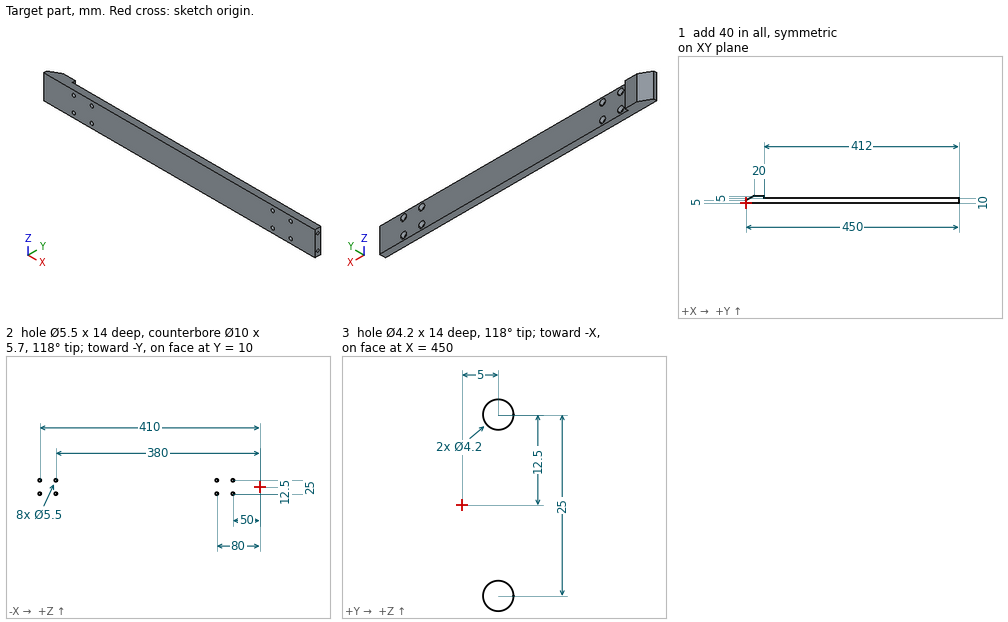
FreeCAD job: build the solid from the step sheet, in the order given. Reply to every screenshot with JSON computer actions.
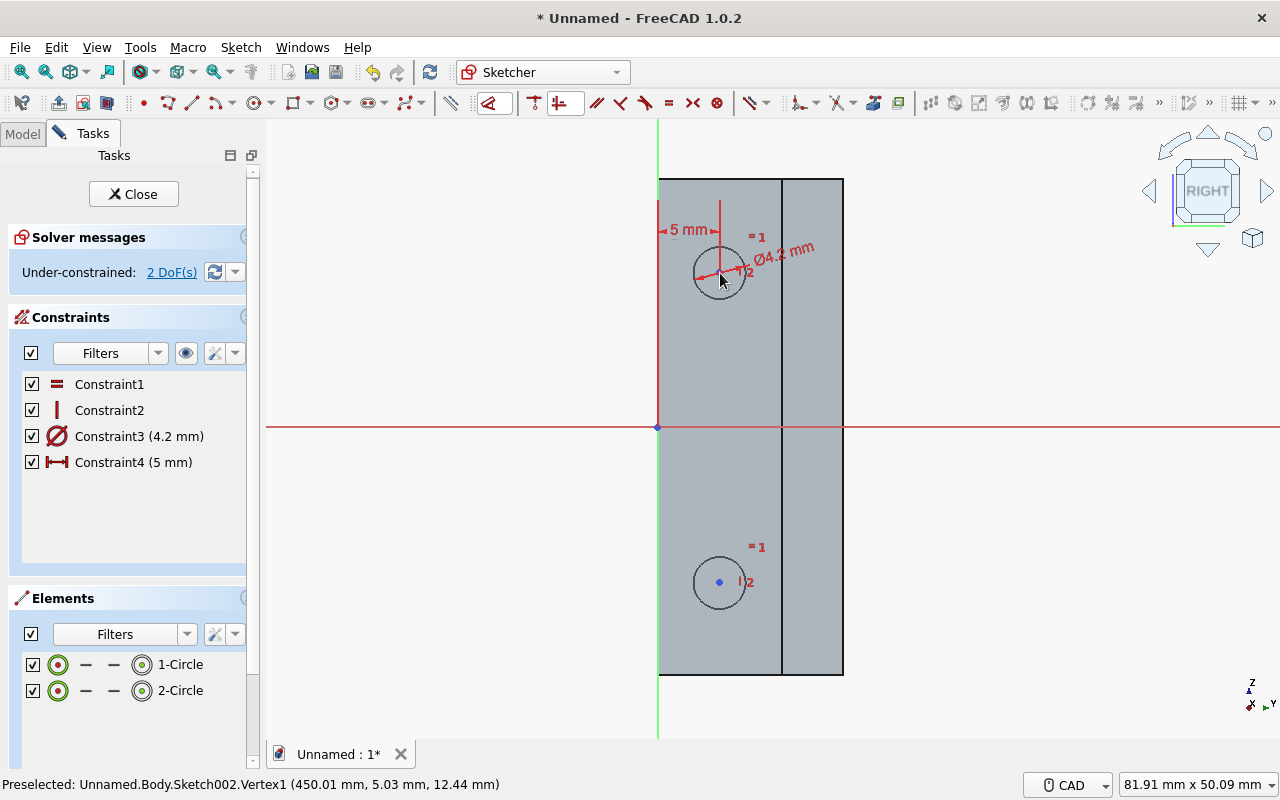
{"action": "left_click", "coordinate": [720, 273]}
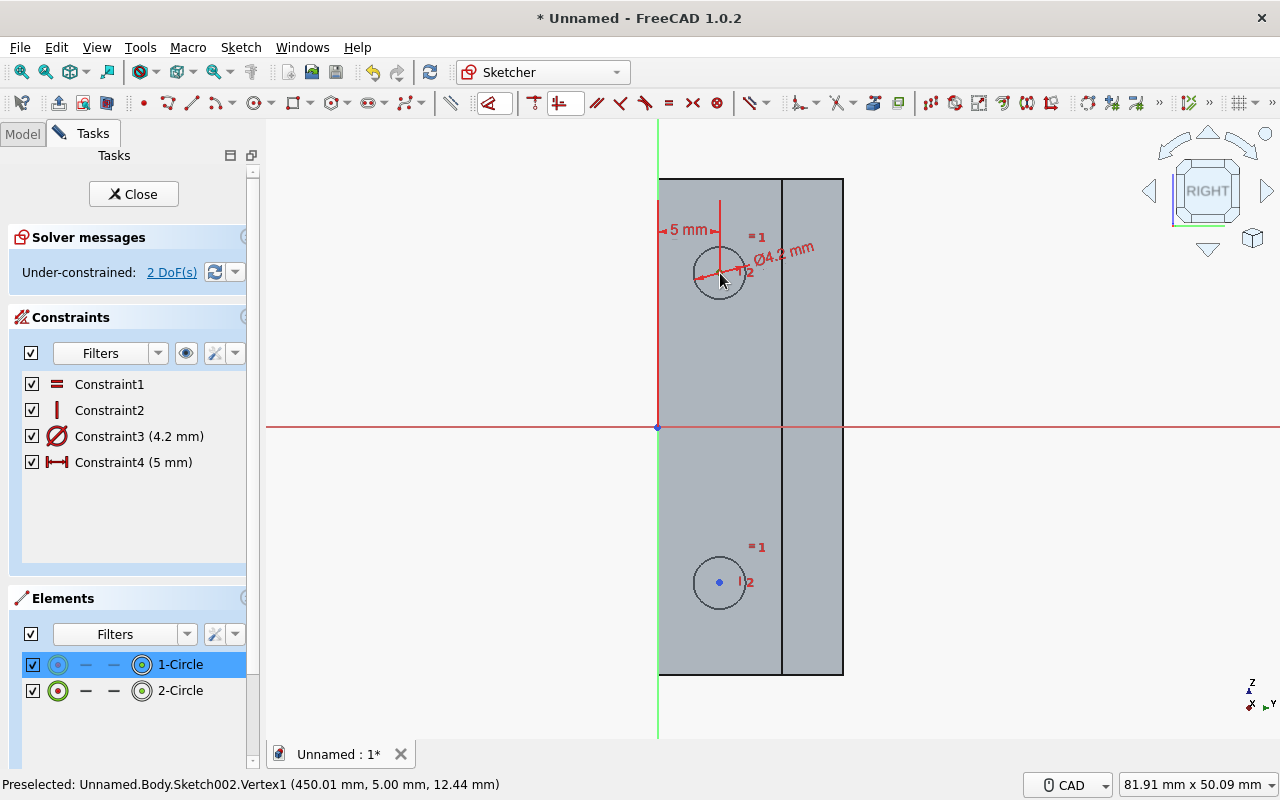
{"action": "left_click", "coordinate": [720, 583]}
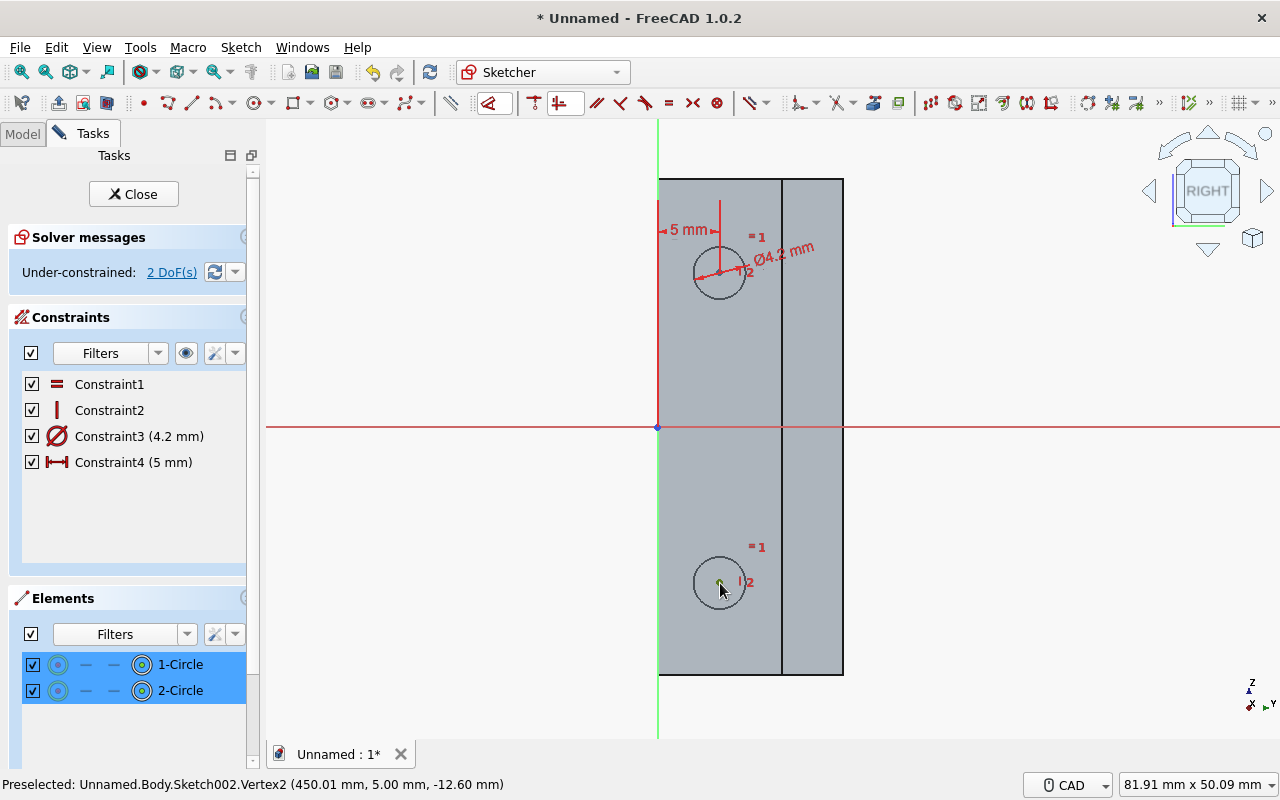
{"action": "left_click", "coordinate": [506, 104]}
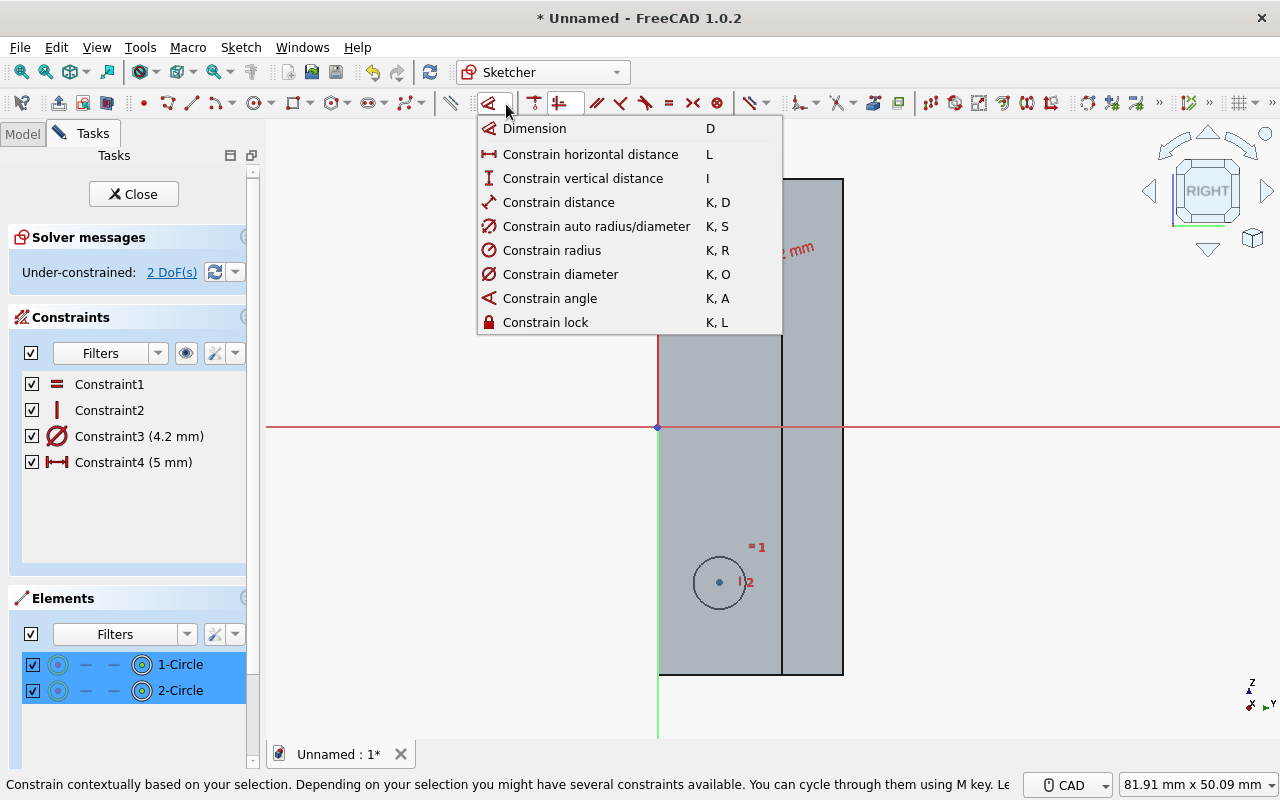
{"action": "left_click", "coordinate": [630, 178]}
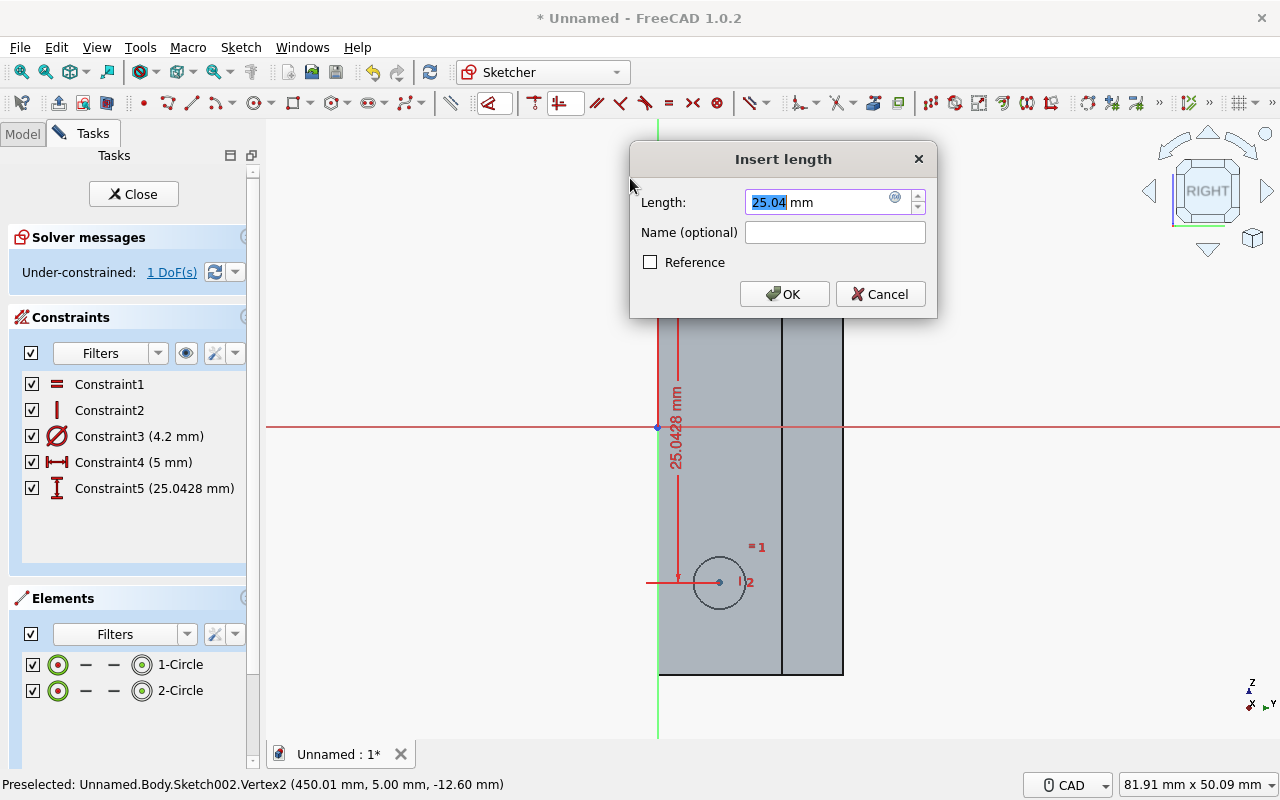
{"action": "type", "text": "25"}
{"action": "key", "text": "Return"}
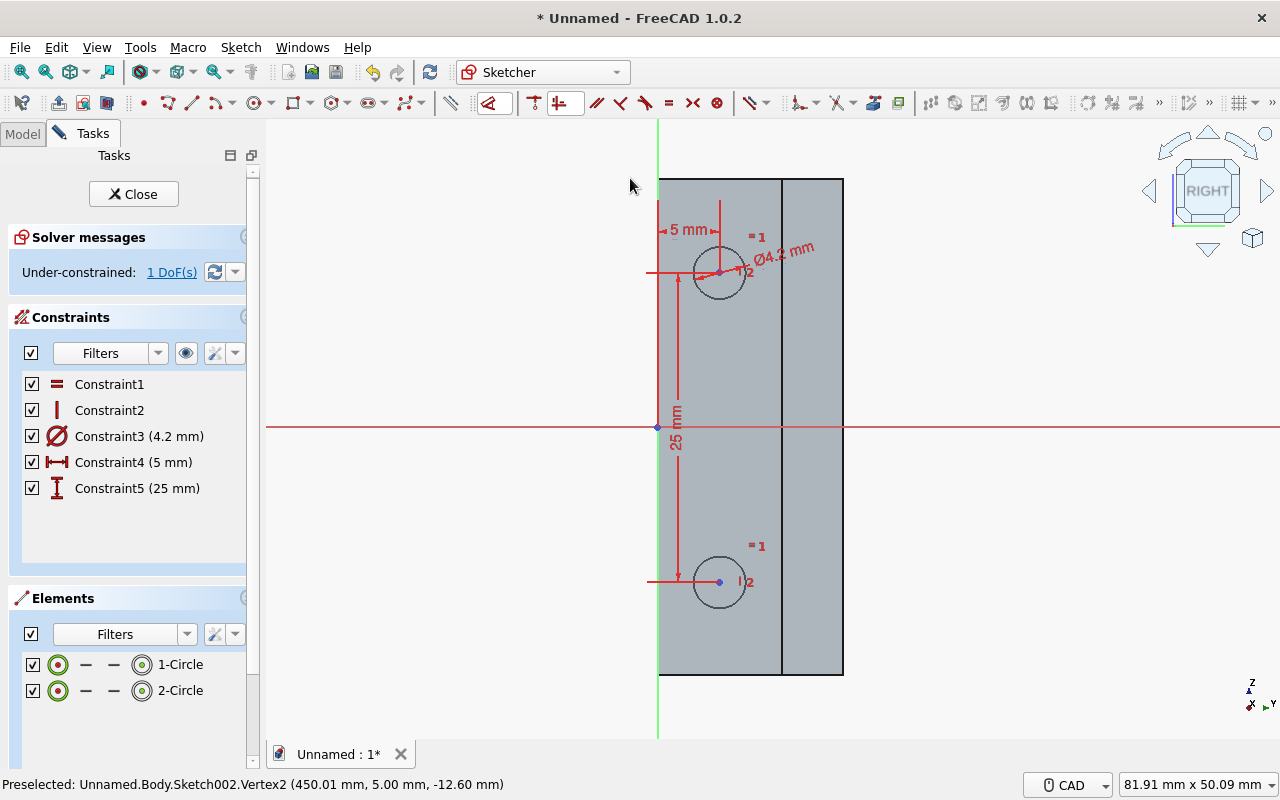
{"action": "left_click", "coordinate": [720, 273]}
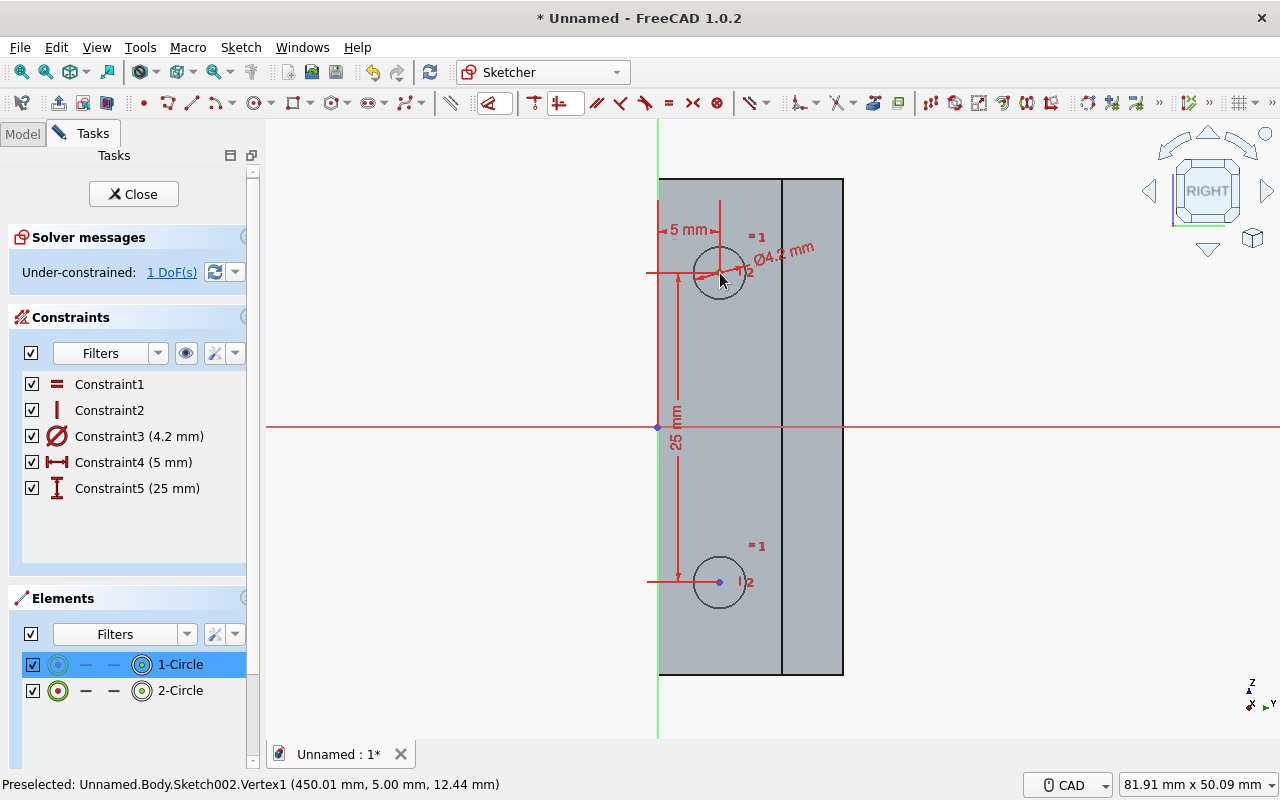
{"action": "key", "text": "i"}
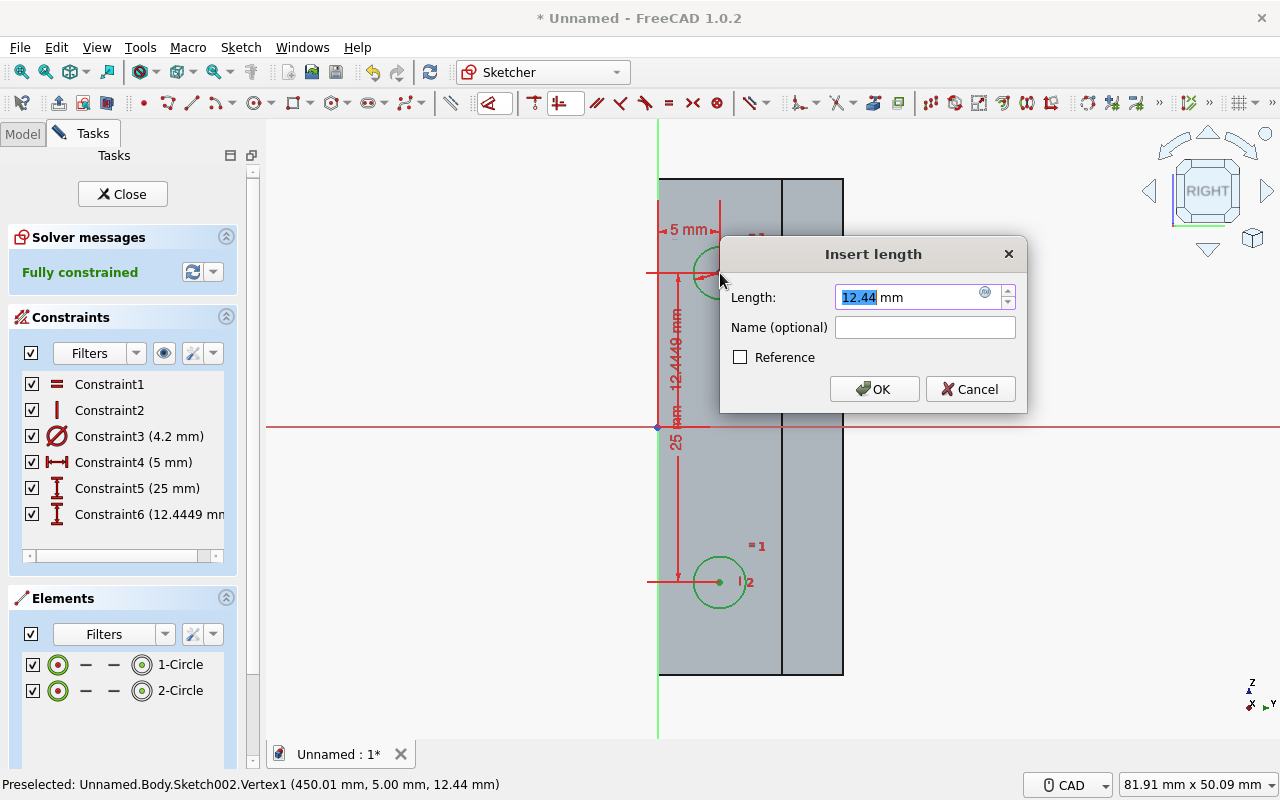
{"action": "type", "text": "12.5"}
{"action": "key", "text": "Return"}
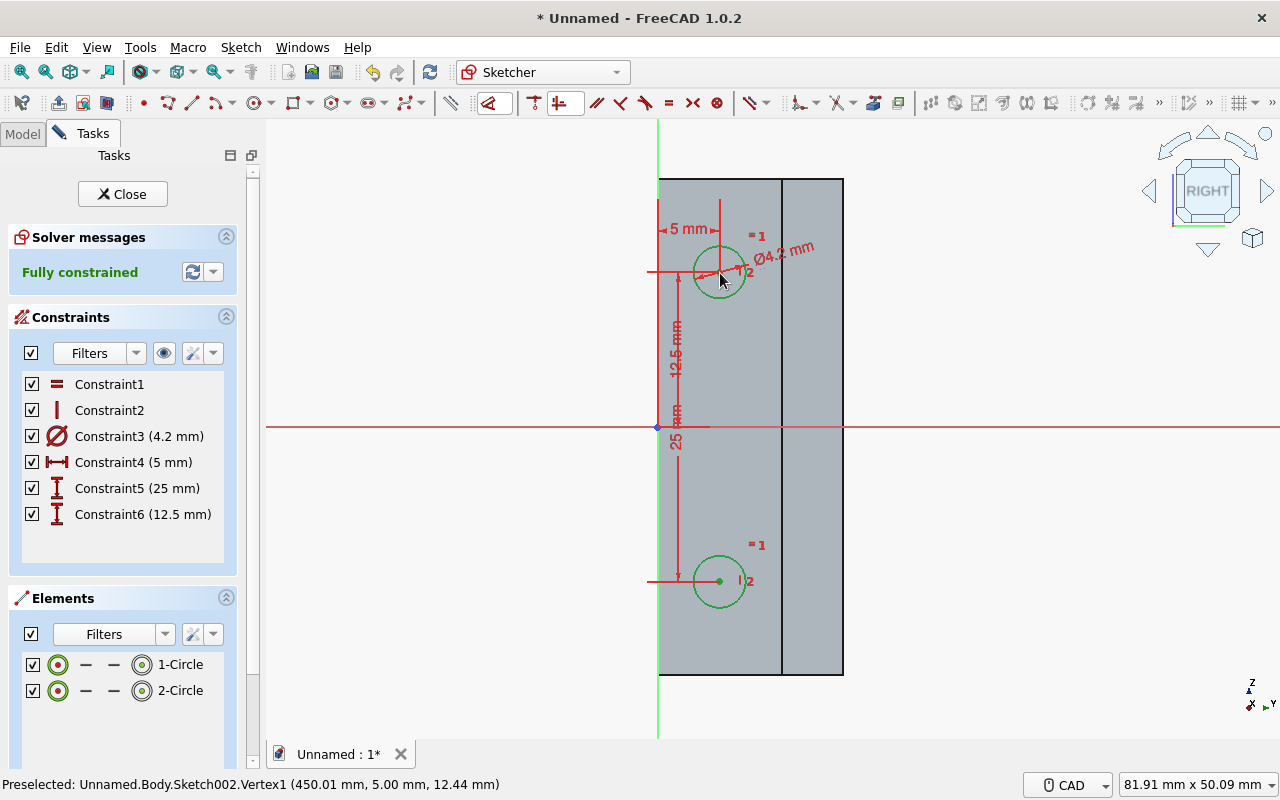
{"action": "left_click", "coordinate": [123, 194]}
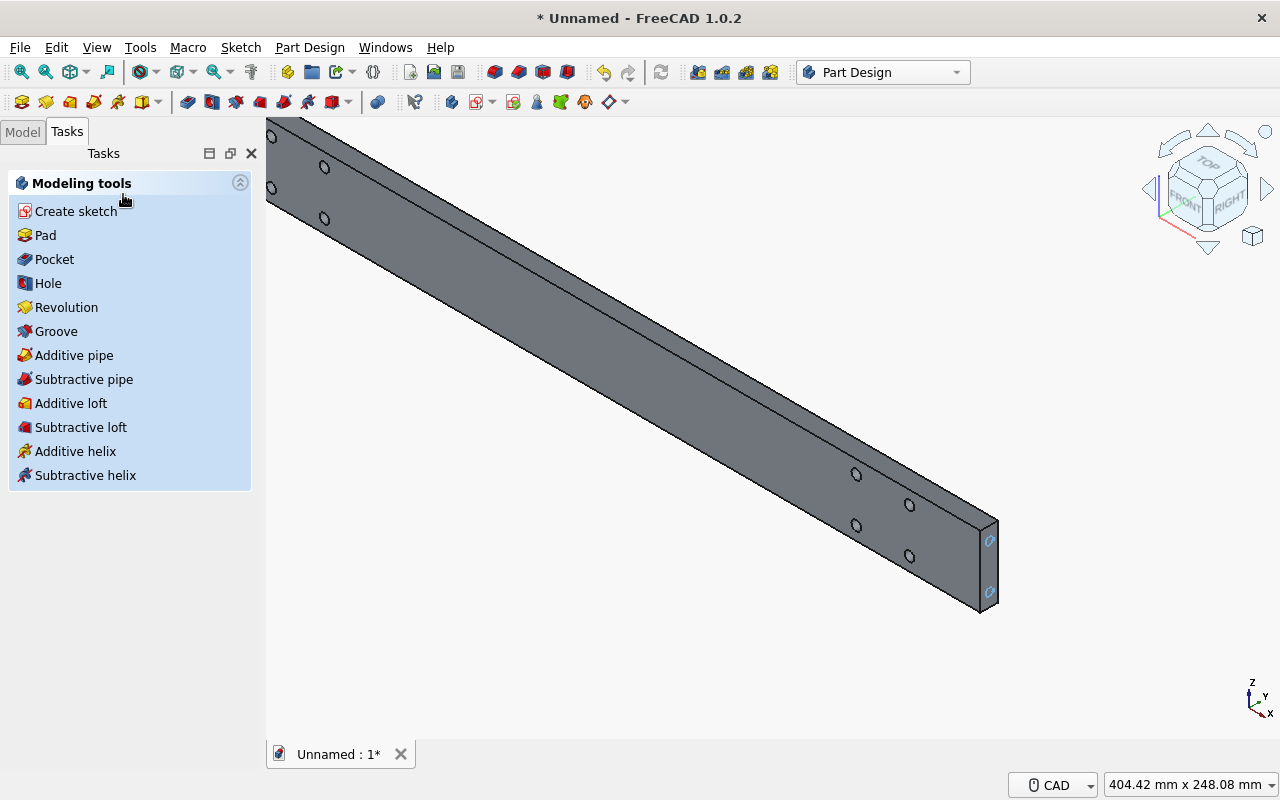
{"action": "left_click", "coordinate": [212, 102]}